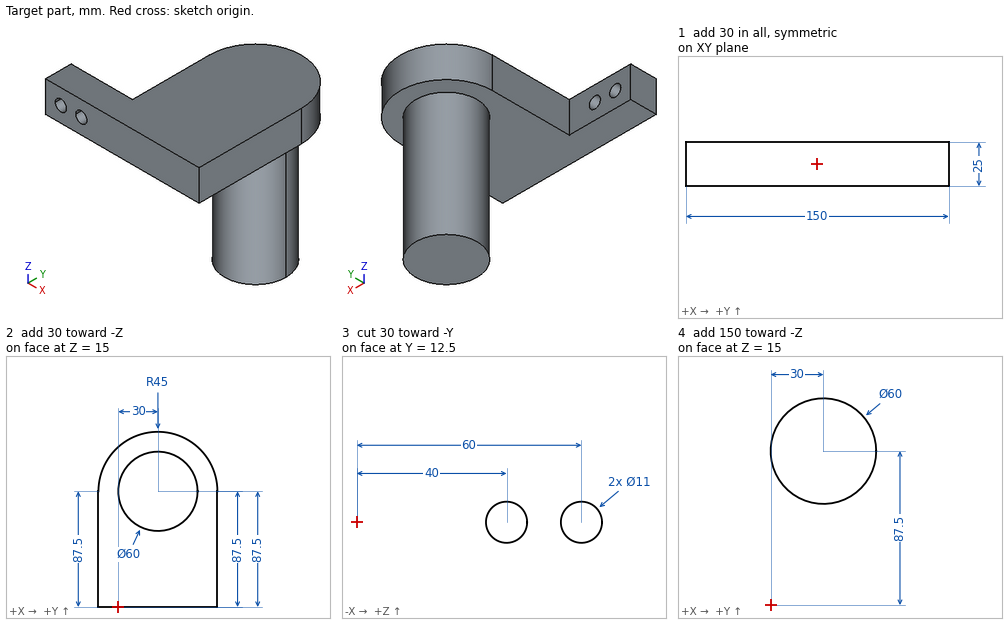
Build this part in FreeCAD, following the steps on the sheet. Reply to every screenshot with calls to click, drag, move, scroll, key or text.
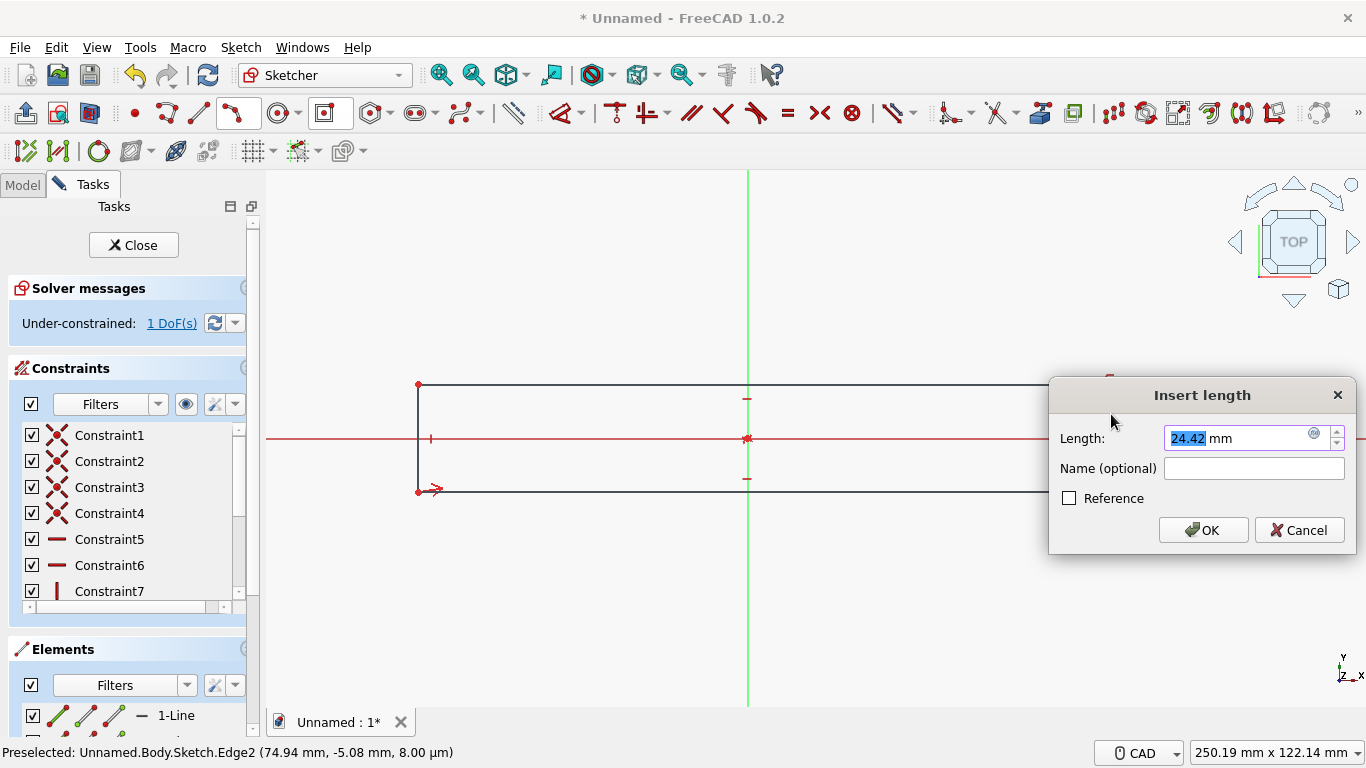
text(25)
key(Return)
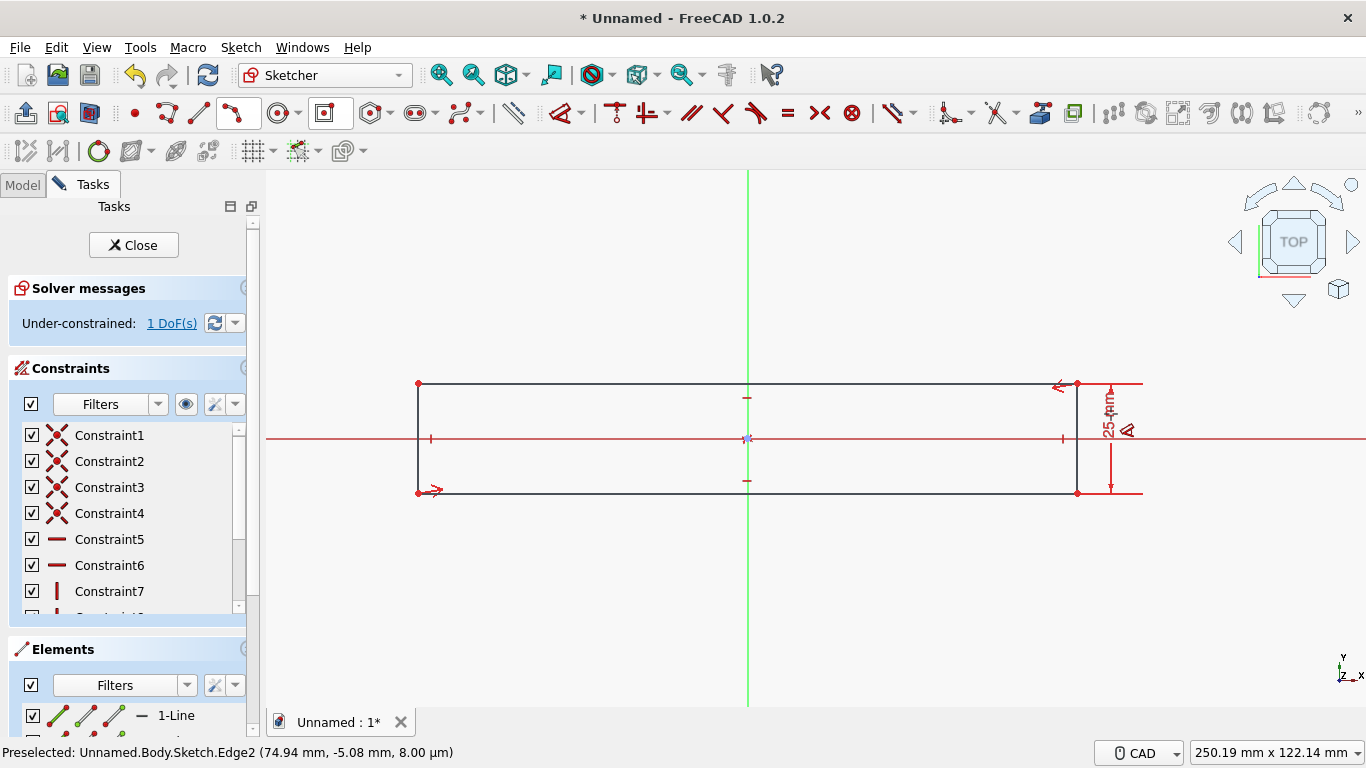
click(616, 494)
click(596, 528)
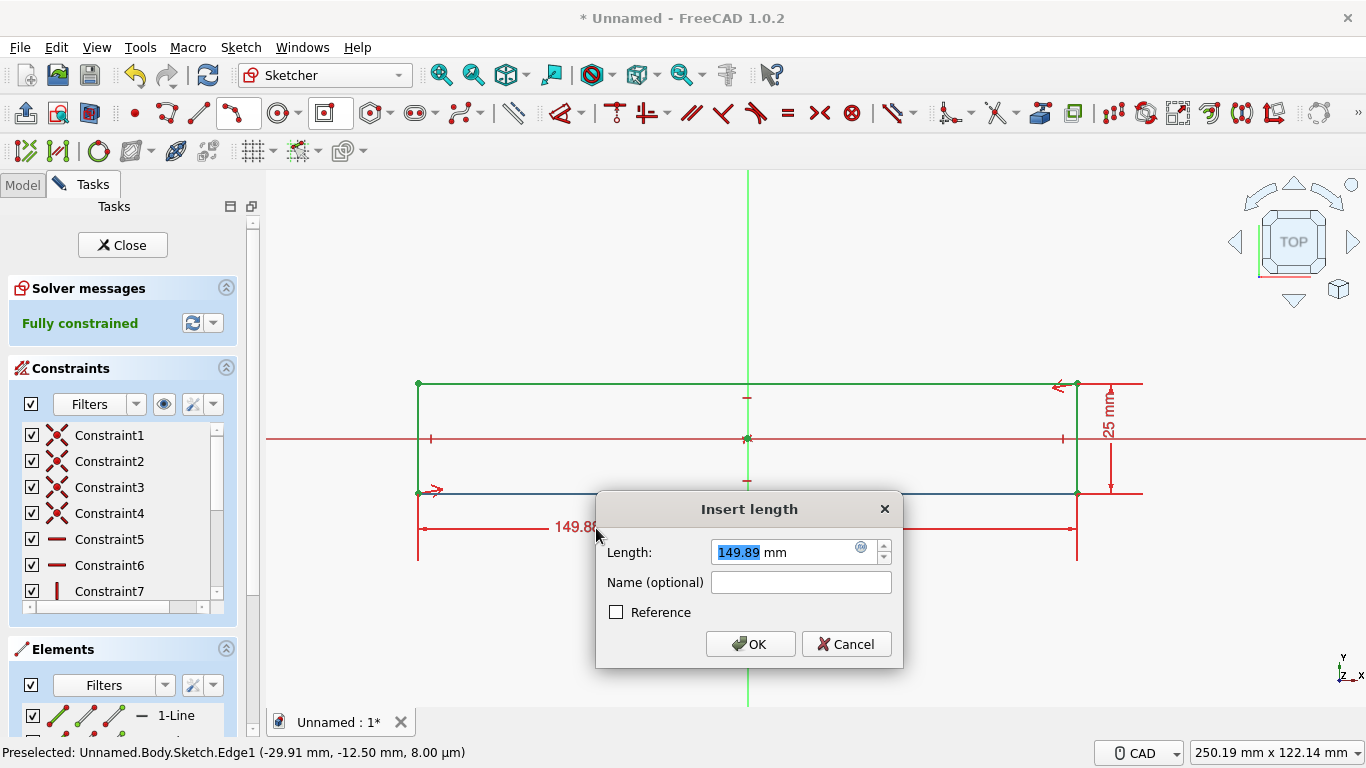
text(150)
key(Return)
key(Escape)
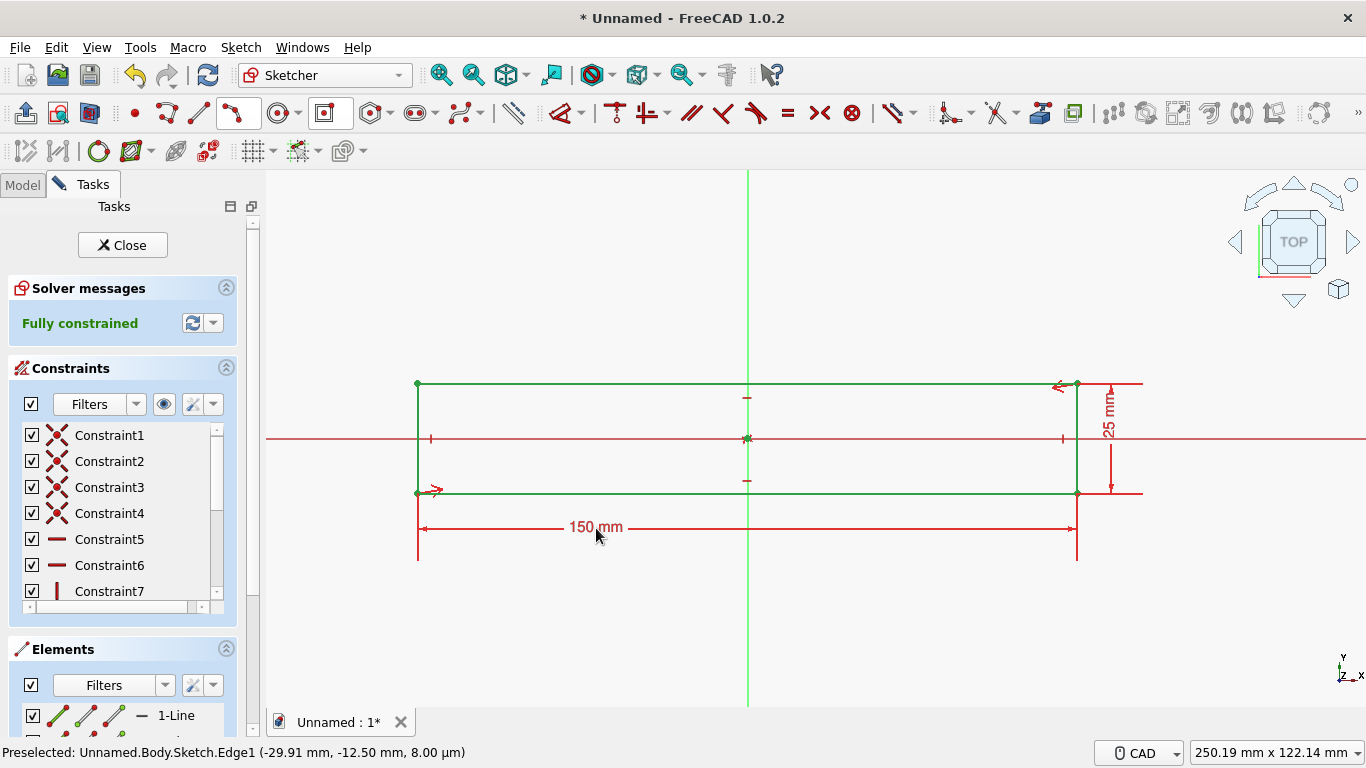
click(123, 245)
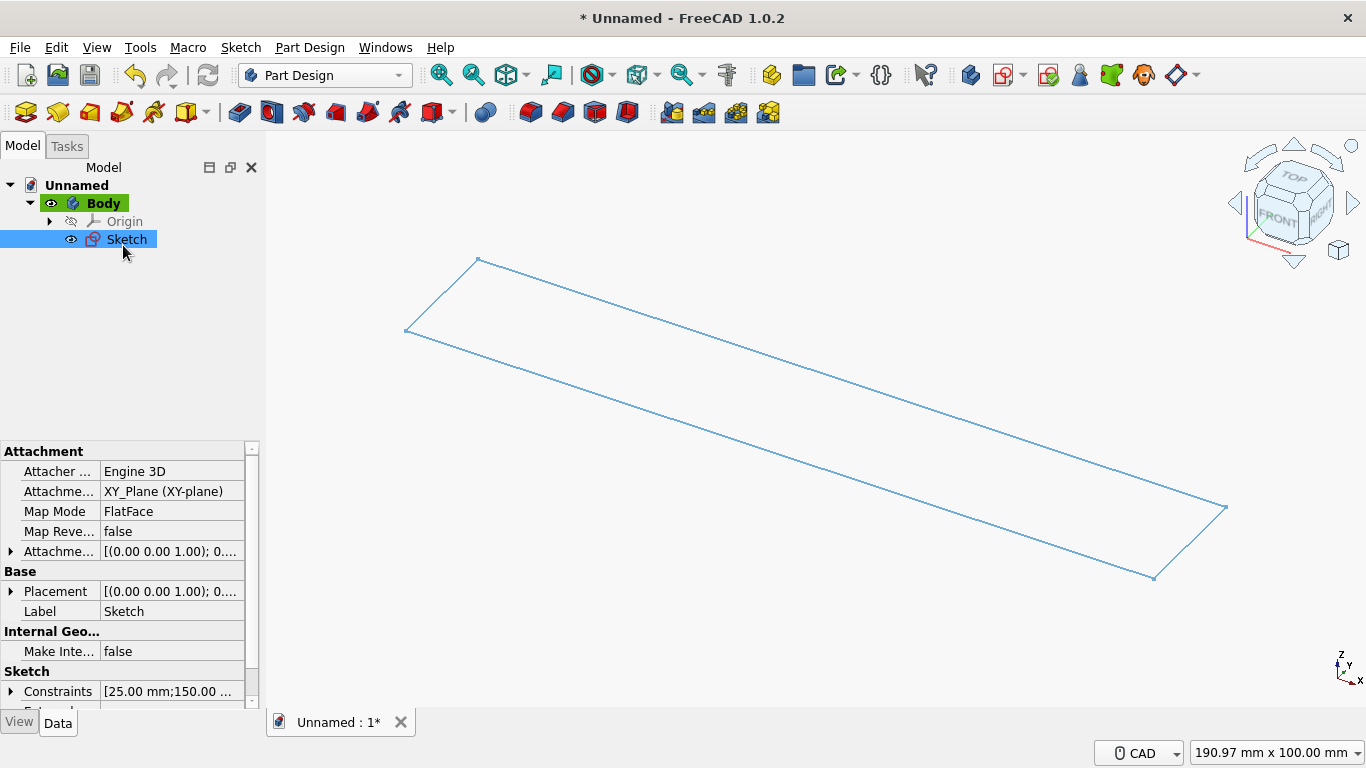
click(26, 112)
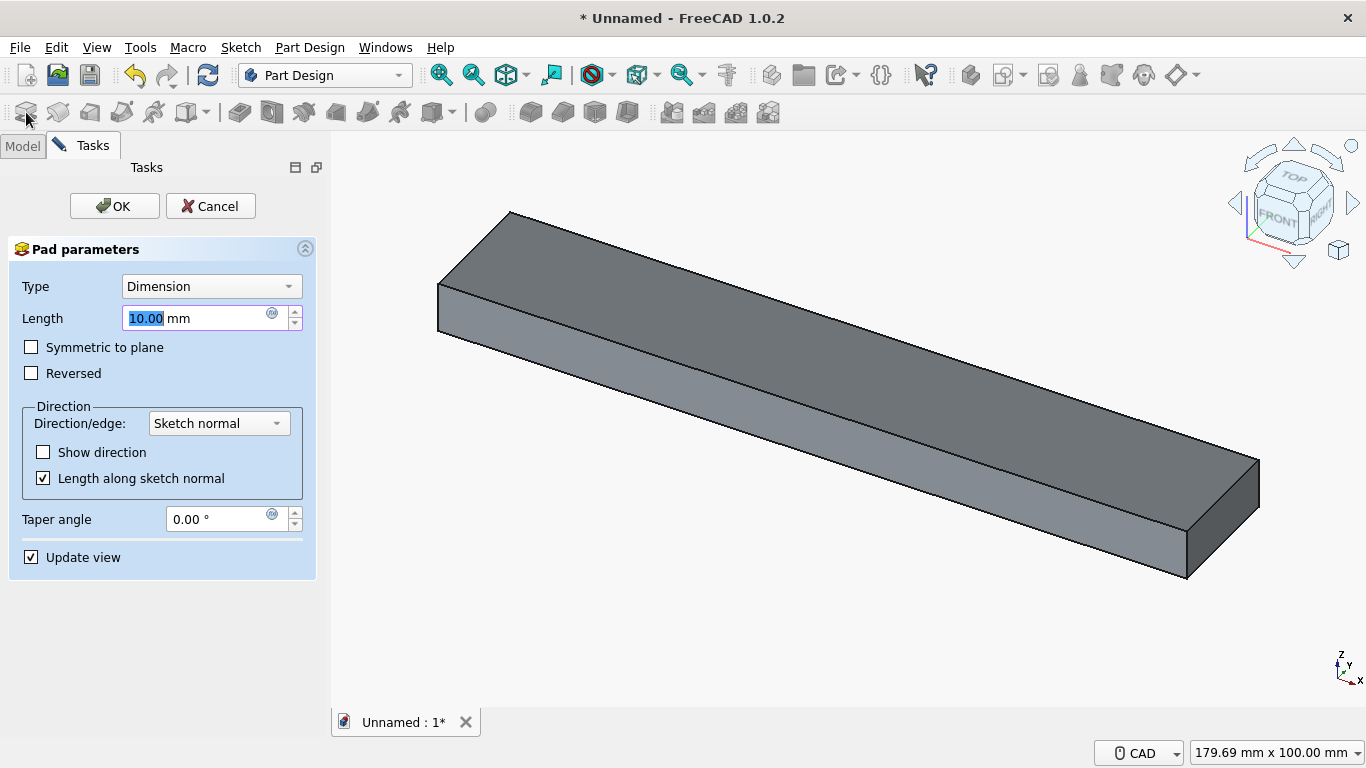
text(30)
key(Tab)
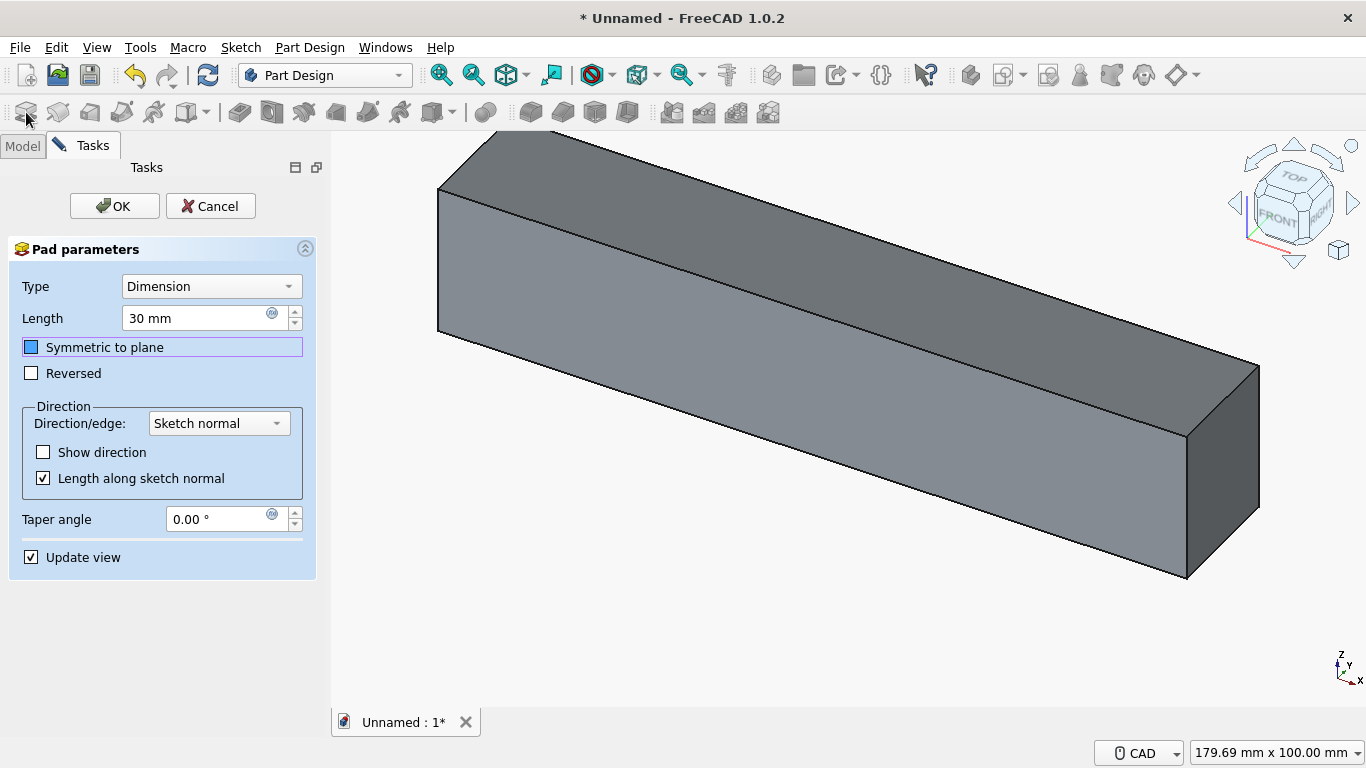
click(30, 347)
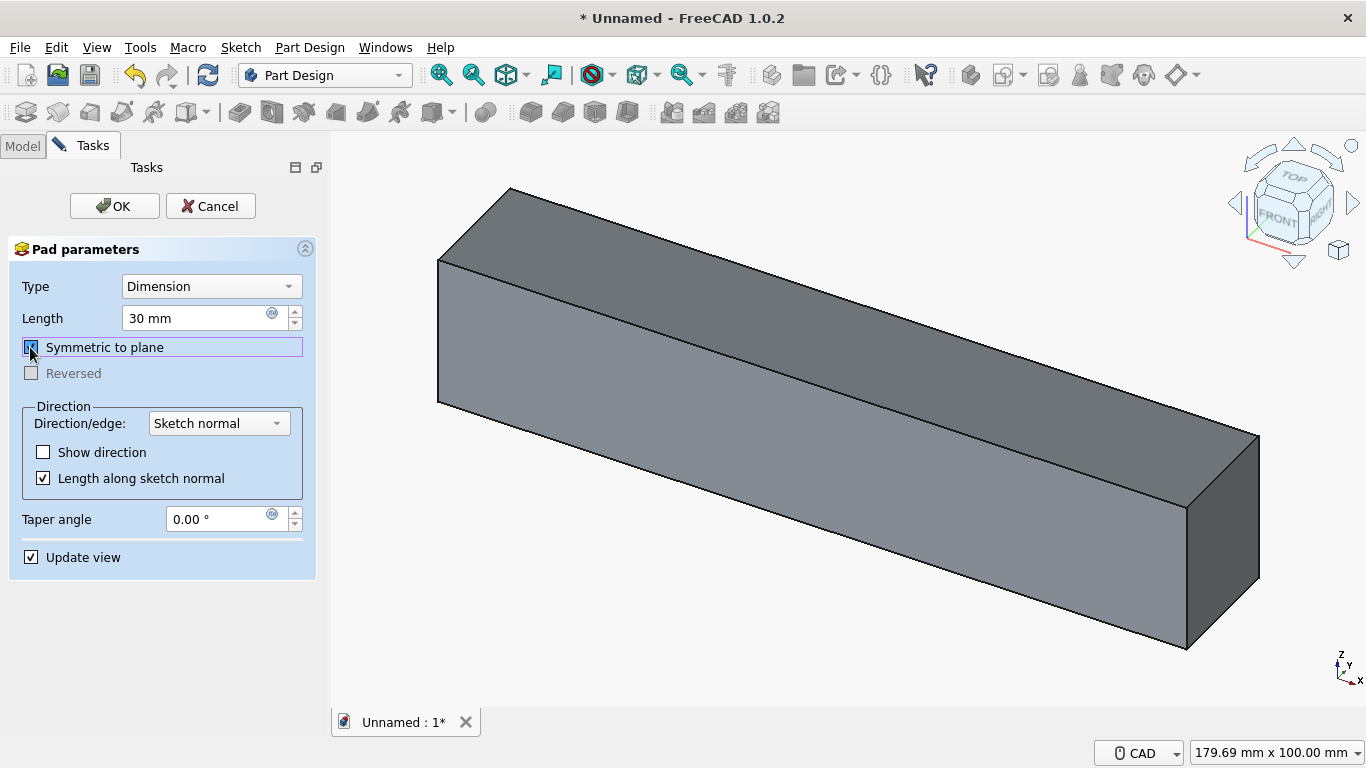
click(115, 206)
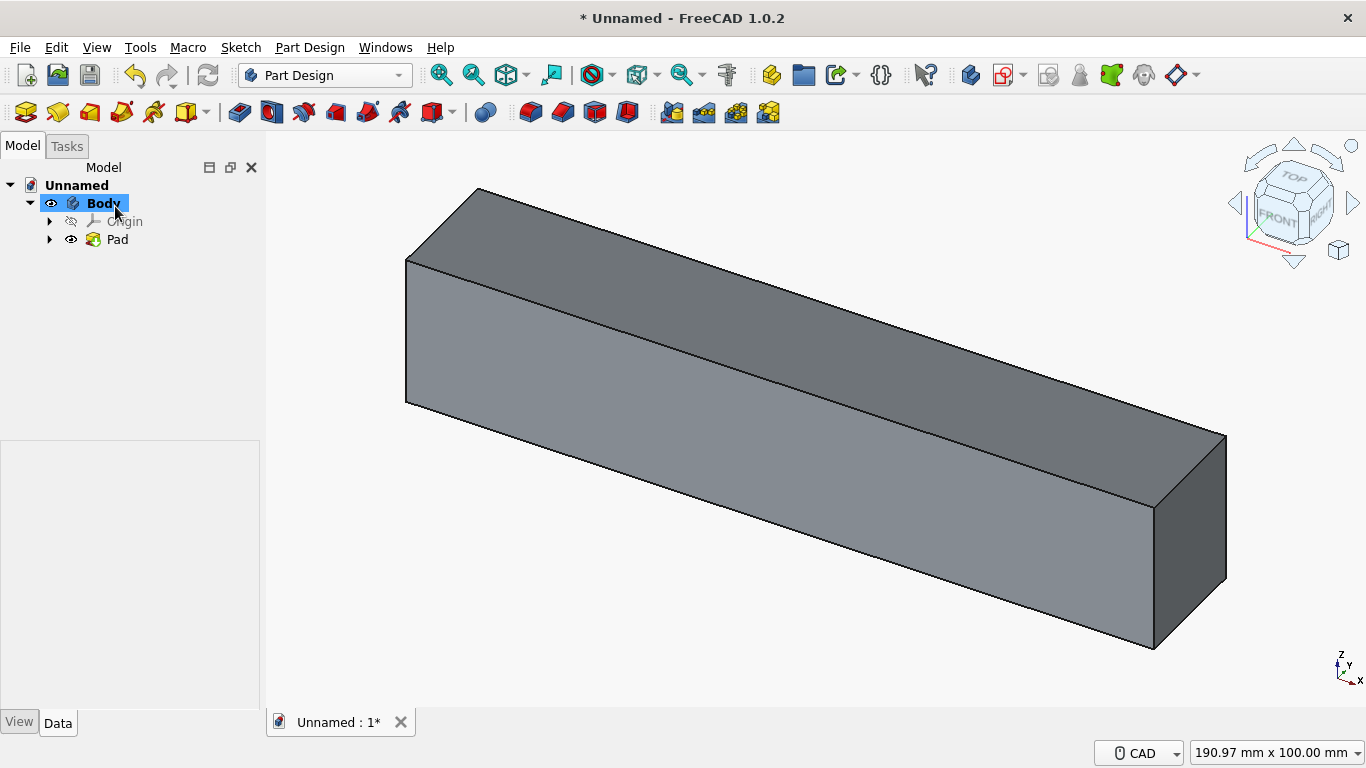
click(1030, 418)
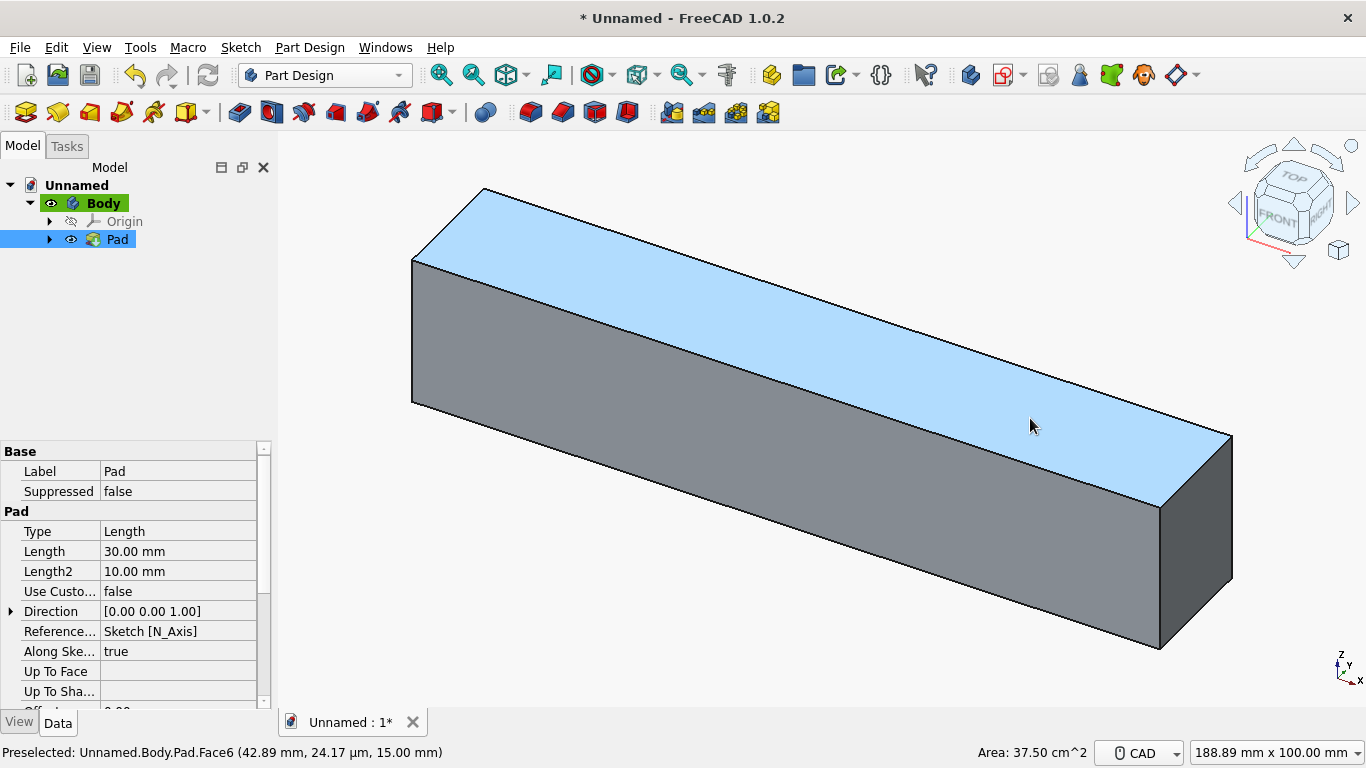
click(1004, 76)